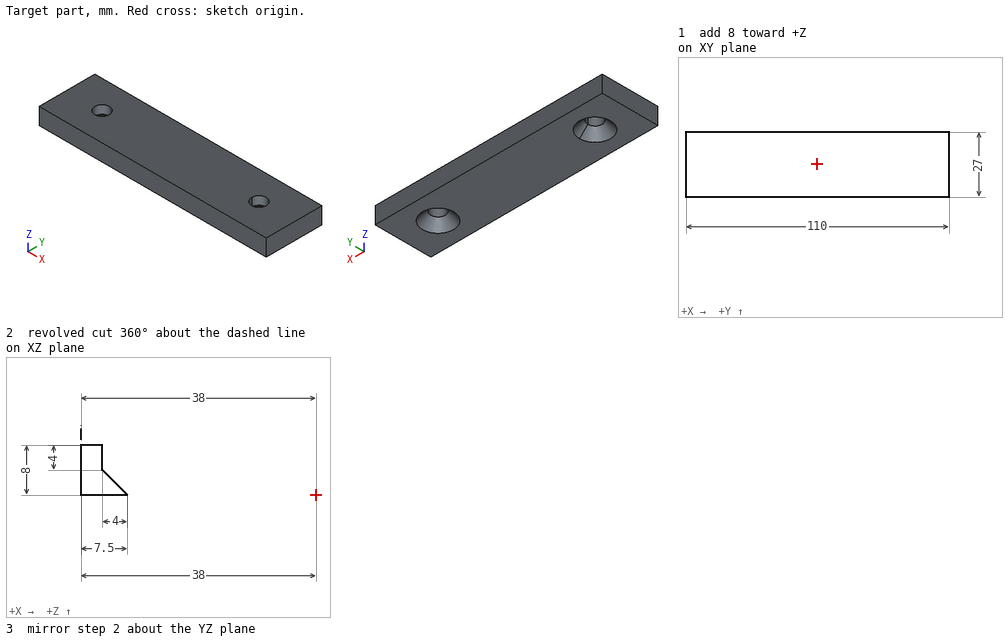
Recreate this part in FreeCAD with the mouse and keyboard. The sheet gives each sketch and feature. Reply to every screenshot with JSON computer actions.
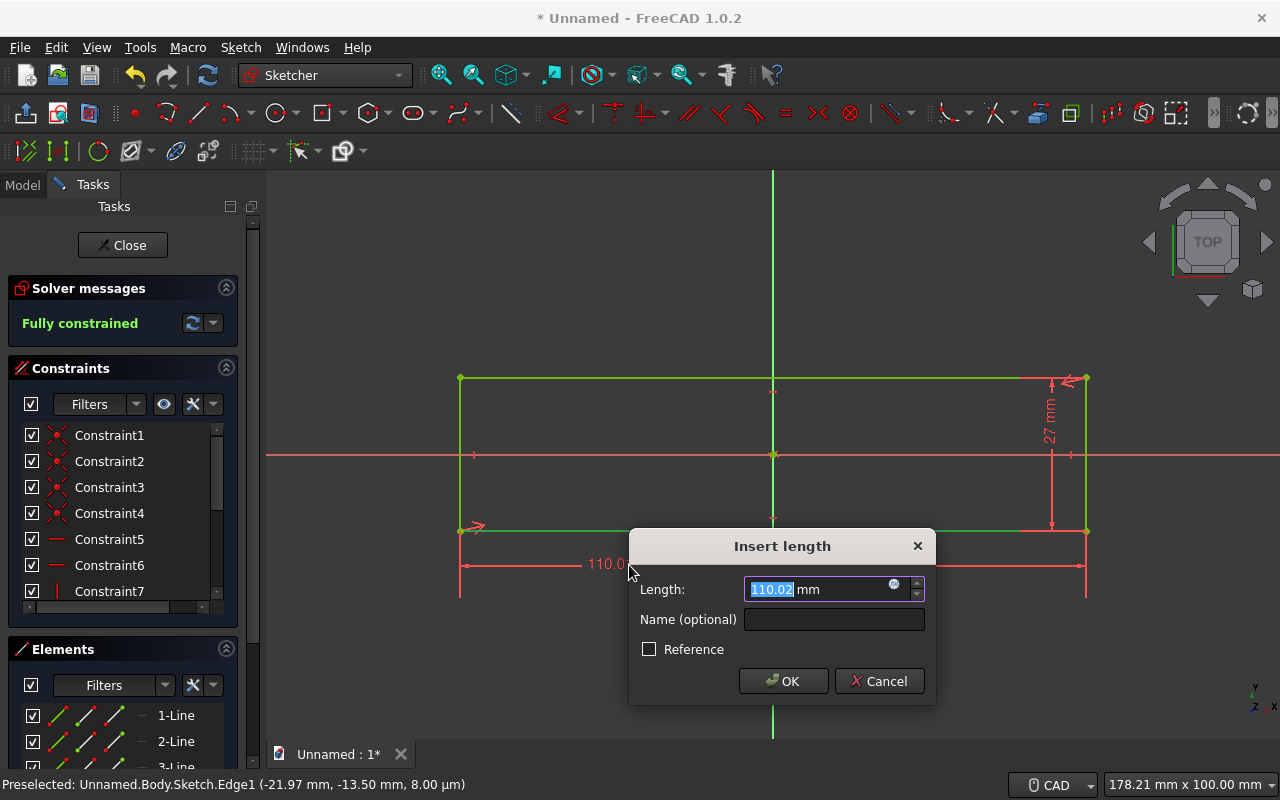
{"action": "type", "text": "110"}
{"action": "key", "text": "Return"}
{"action": "key", "text": "Escape"}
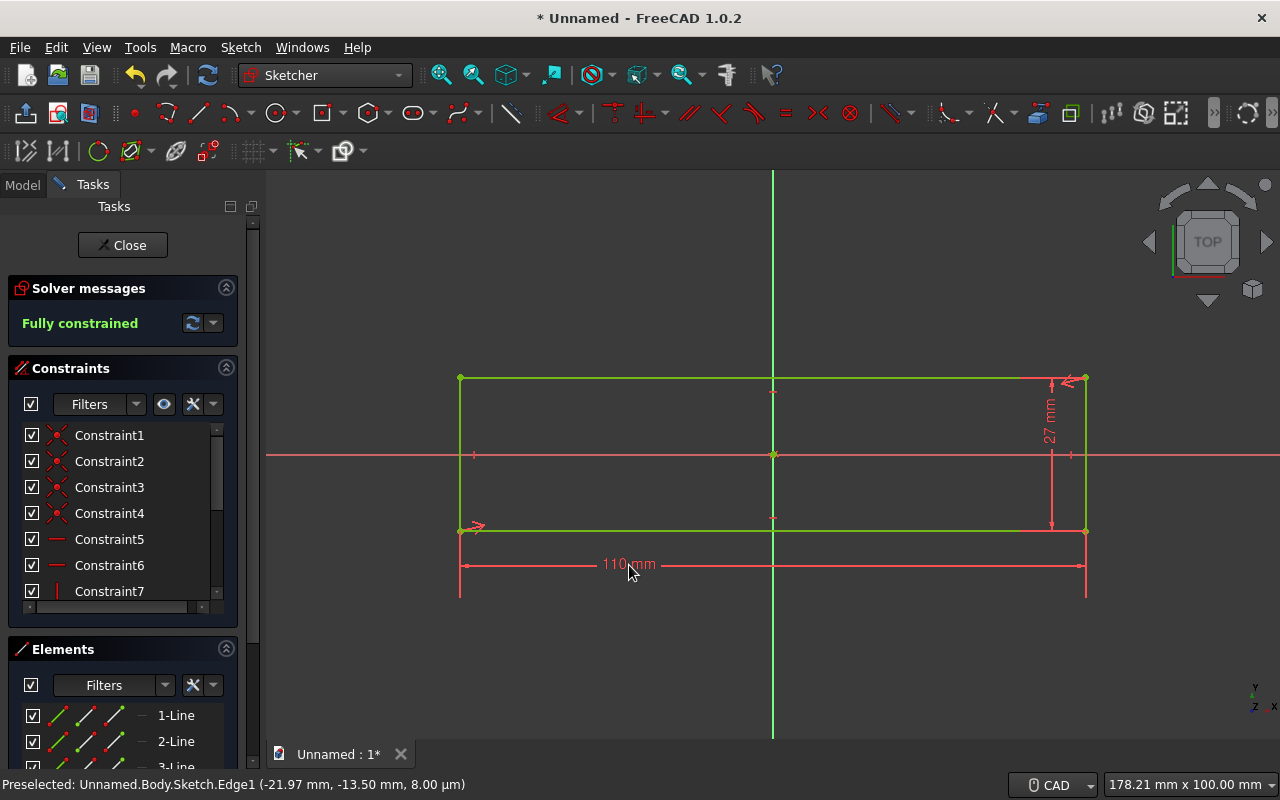
{"action": "left_click", "coordinate": [123, 245]}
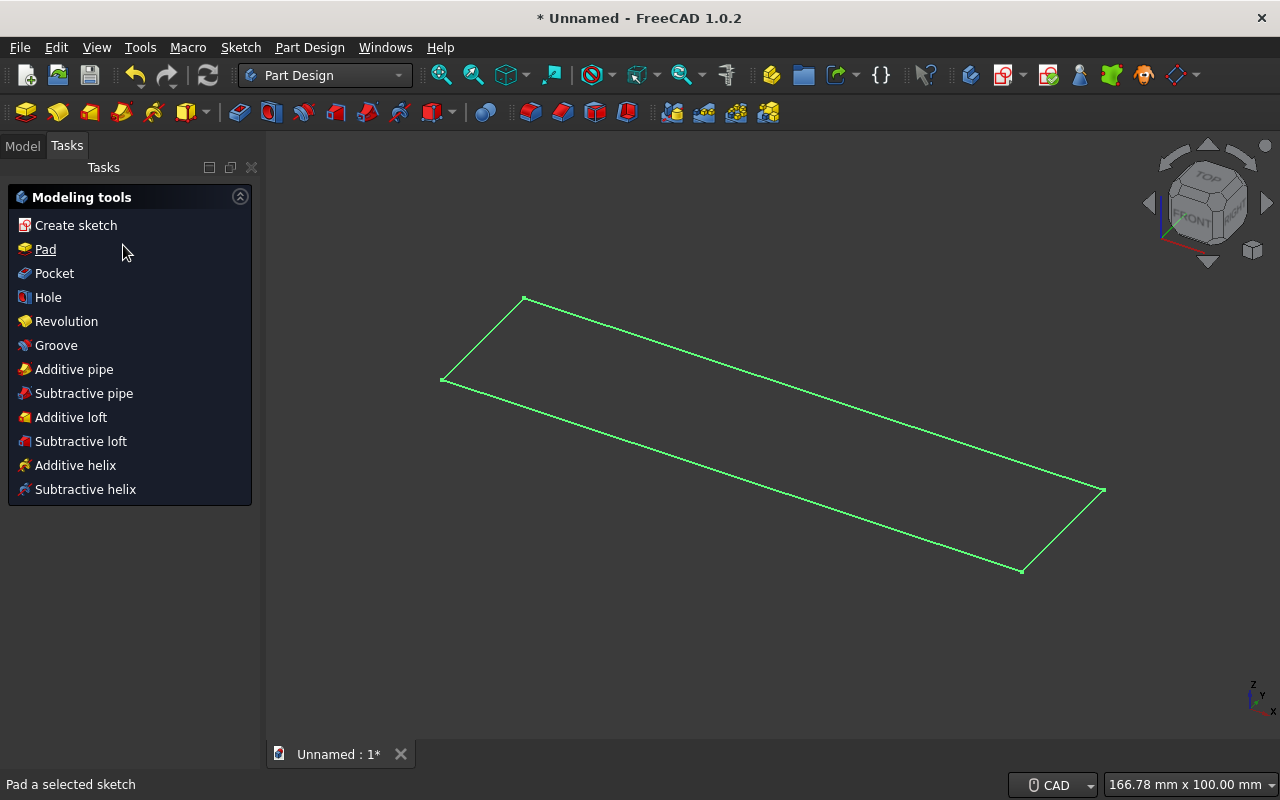
{"action": "left_click", "coordinate": [26, 112]}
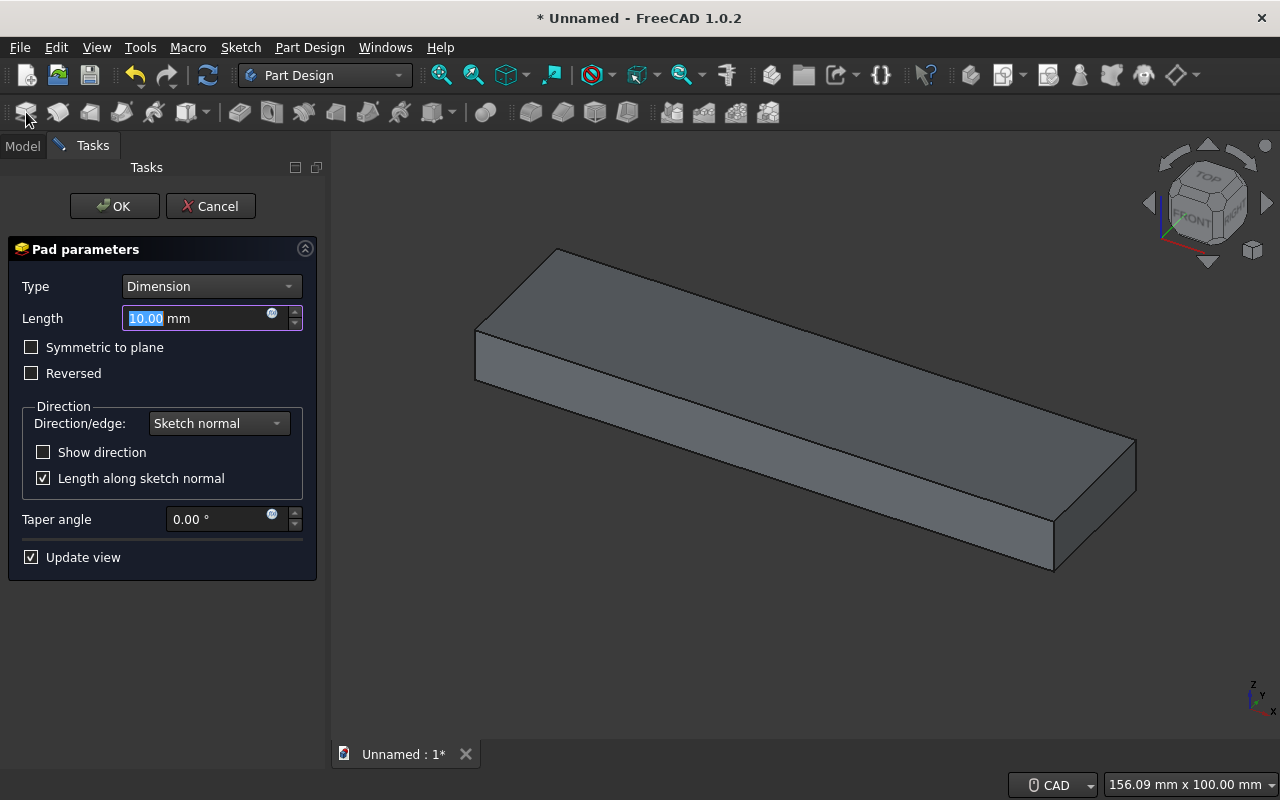
{"action": "type", "text": "8"}
{"action": "key", "text": "Tab"}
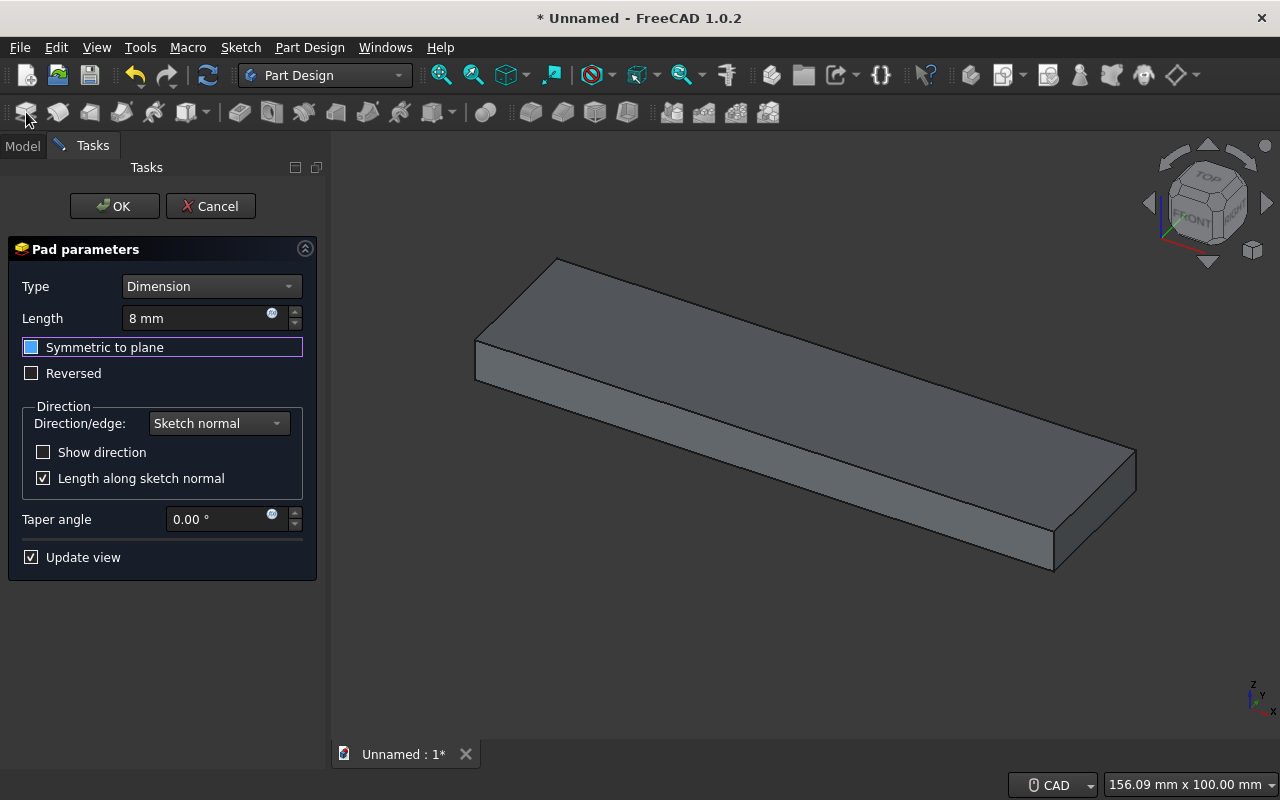
{"action": "left_click", "coordinate": [115, 206]}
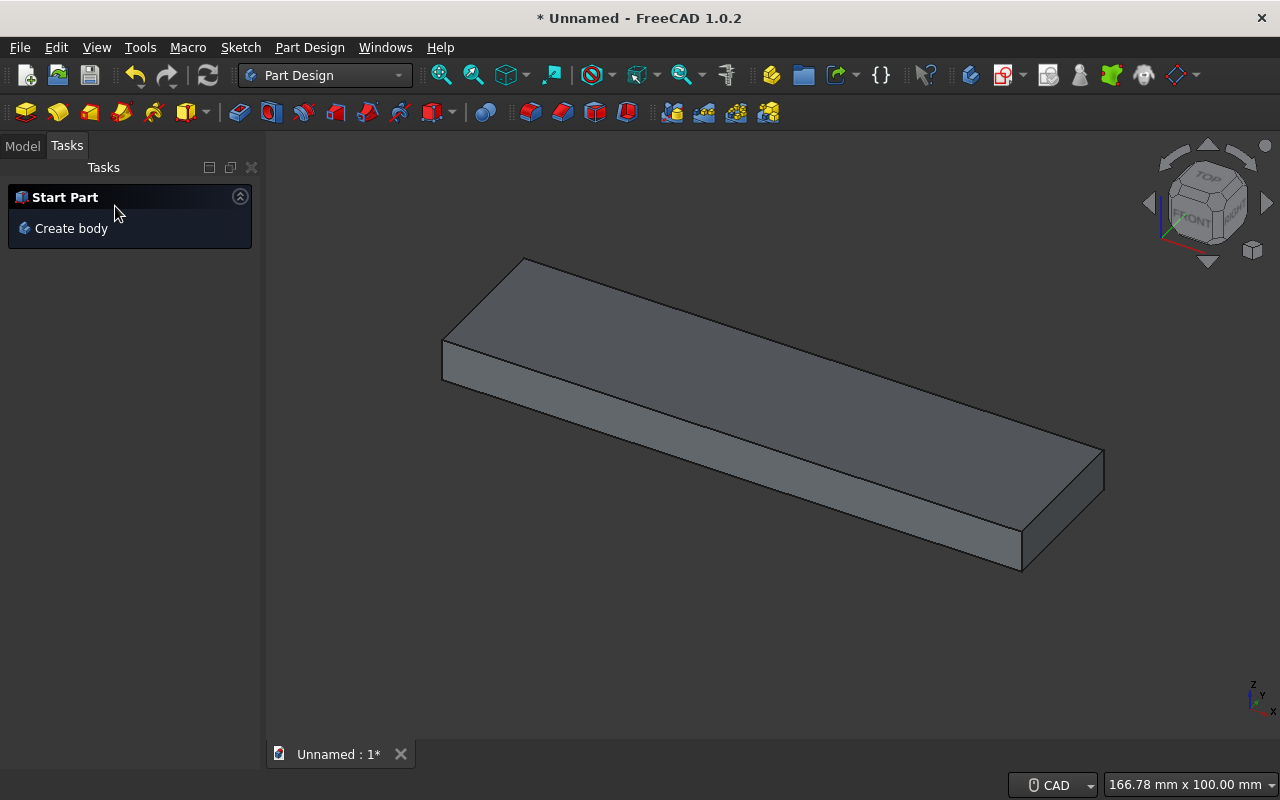
{"action": "left_click", "coordinate": [1004, 76]}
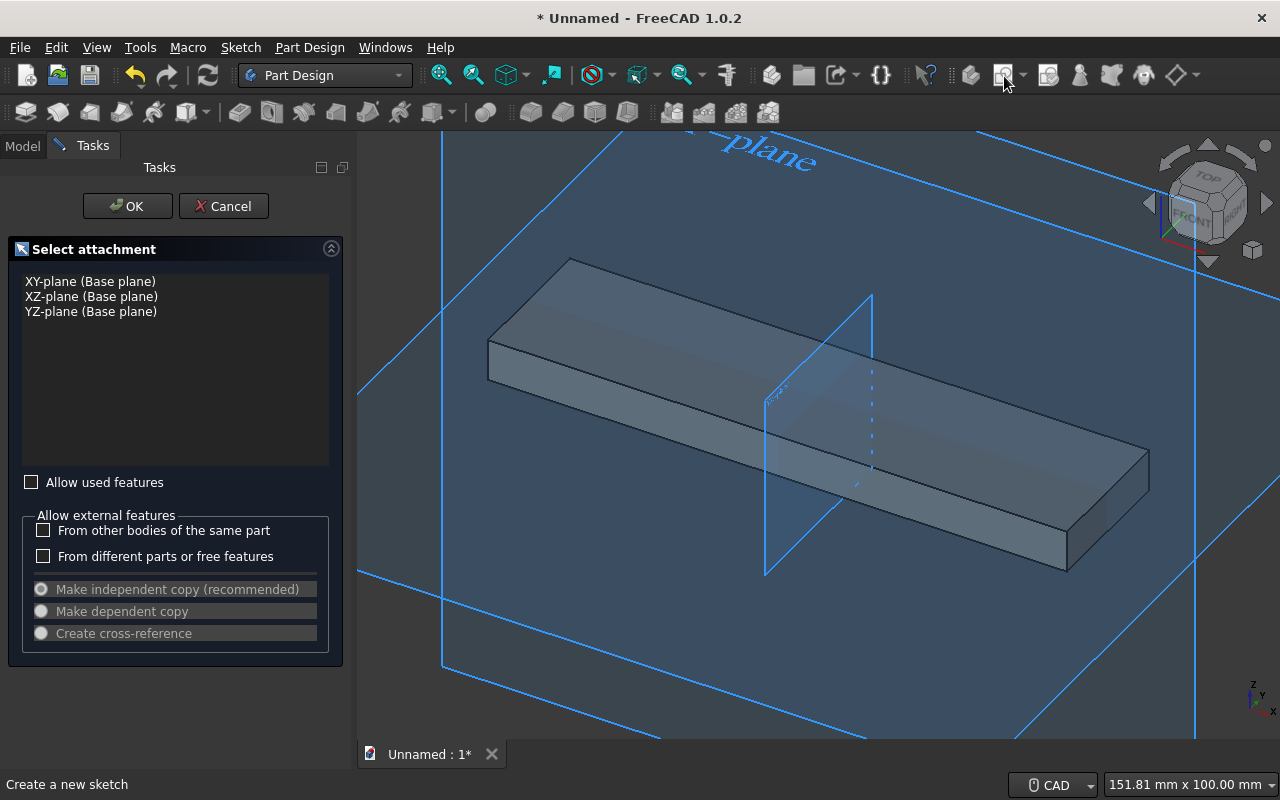
{"action": "left_click", "coordinate": [82, 296]}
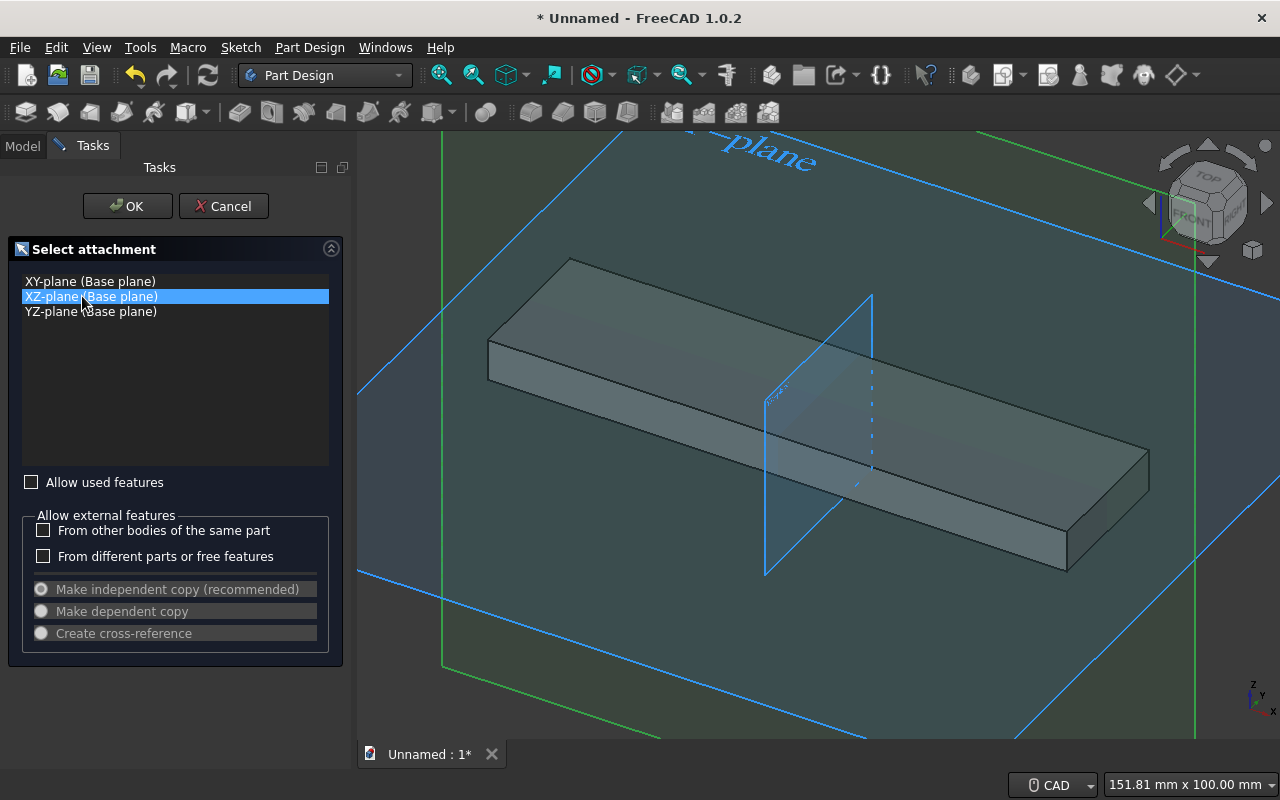
{"action": "left_click", "coordinate": [128, 206]}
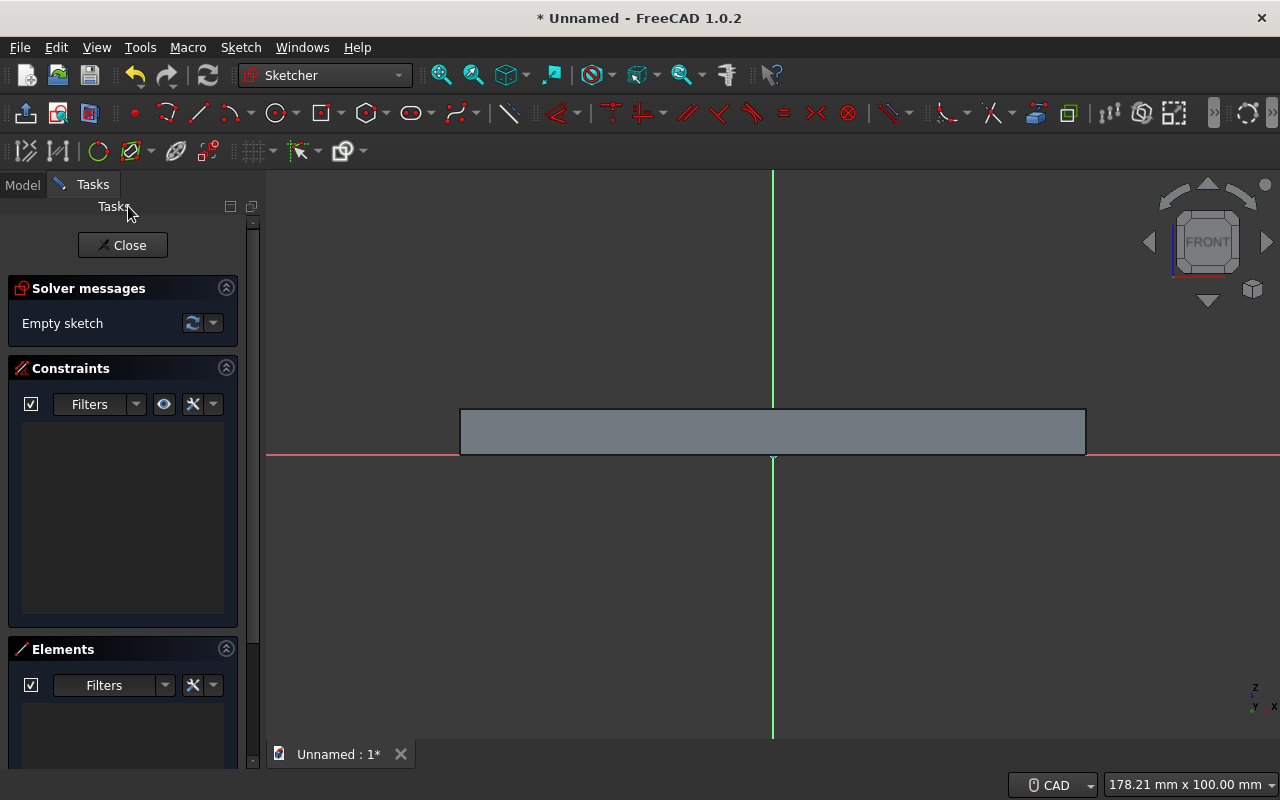
{"action": "left_click", "coordinate": [90, 114]}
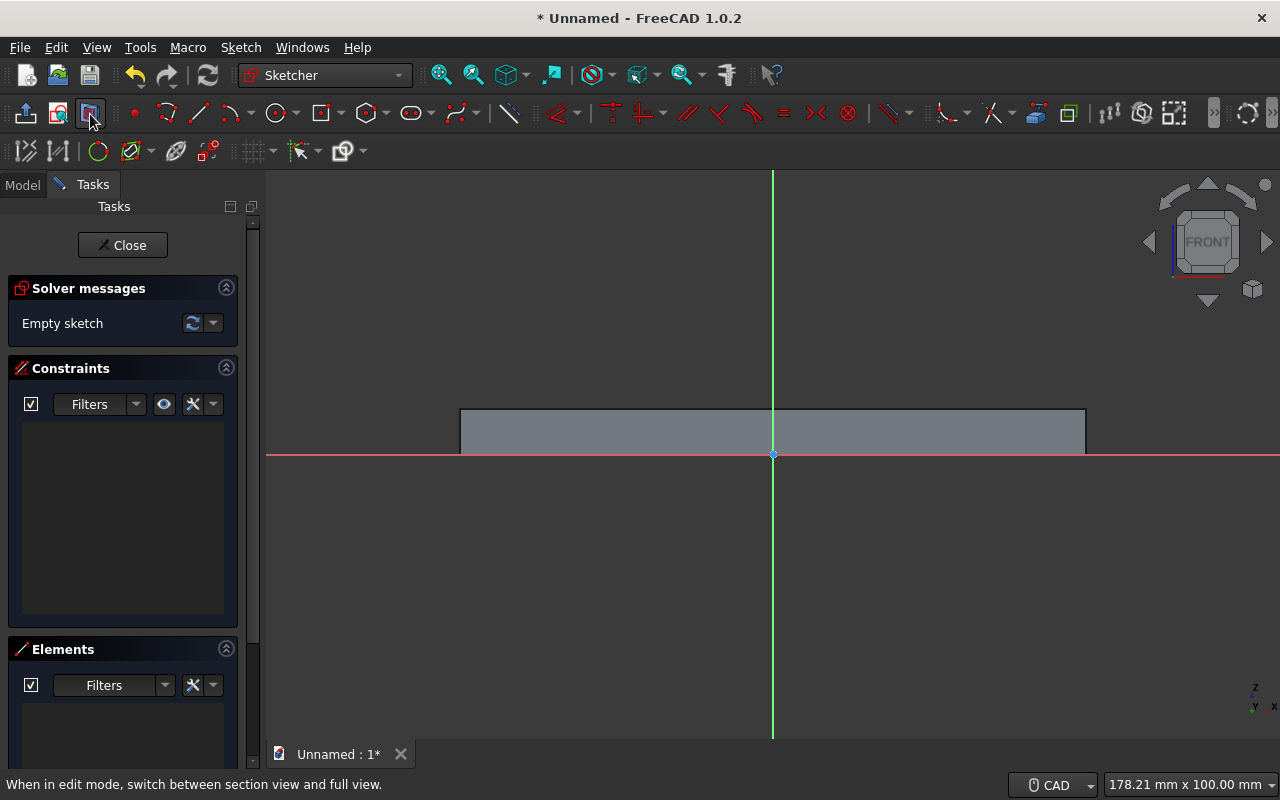
{"action": "scroll", "coordinate": [553, 416], "scroll_direction": "up", "scroll_amount": 9}